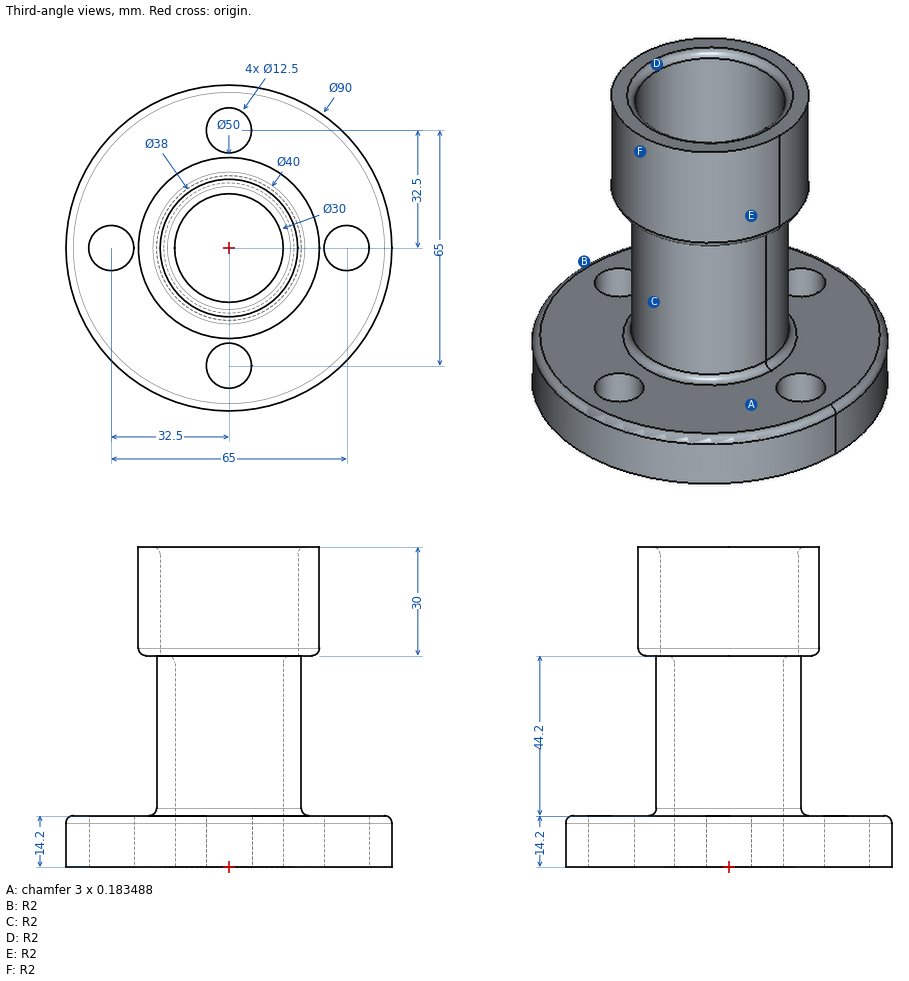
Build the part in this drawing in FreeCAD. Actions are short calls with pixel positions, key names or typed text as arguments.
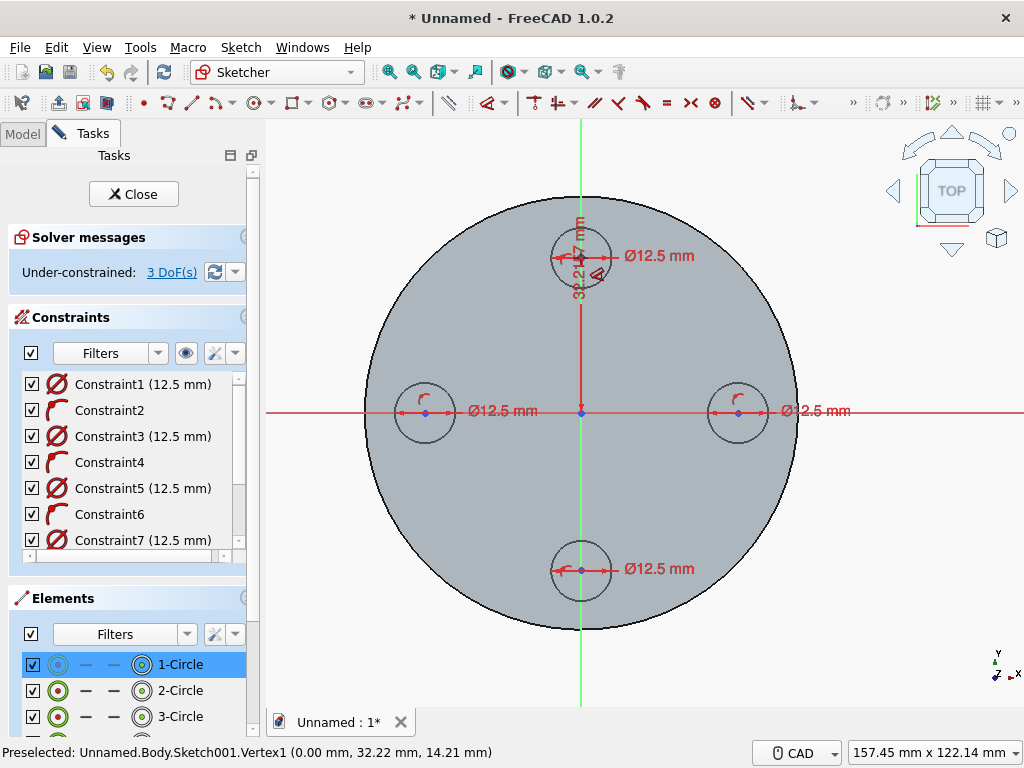
click(581, 571)
click(615, 343)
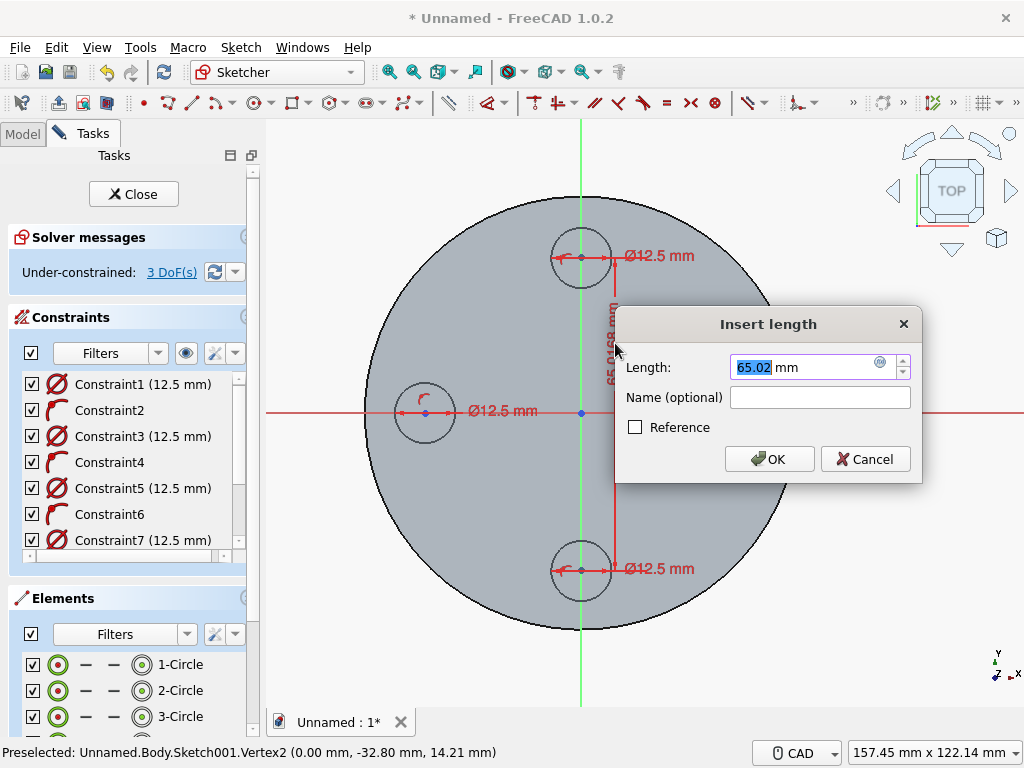
text(65)
key(Return)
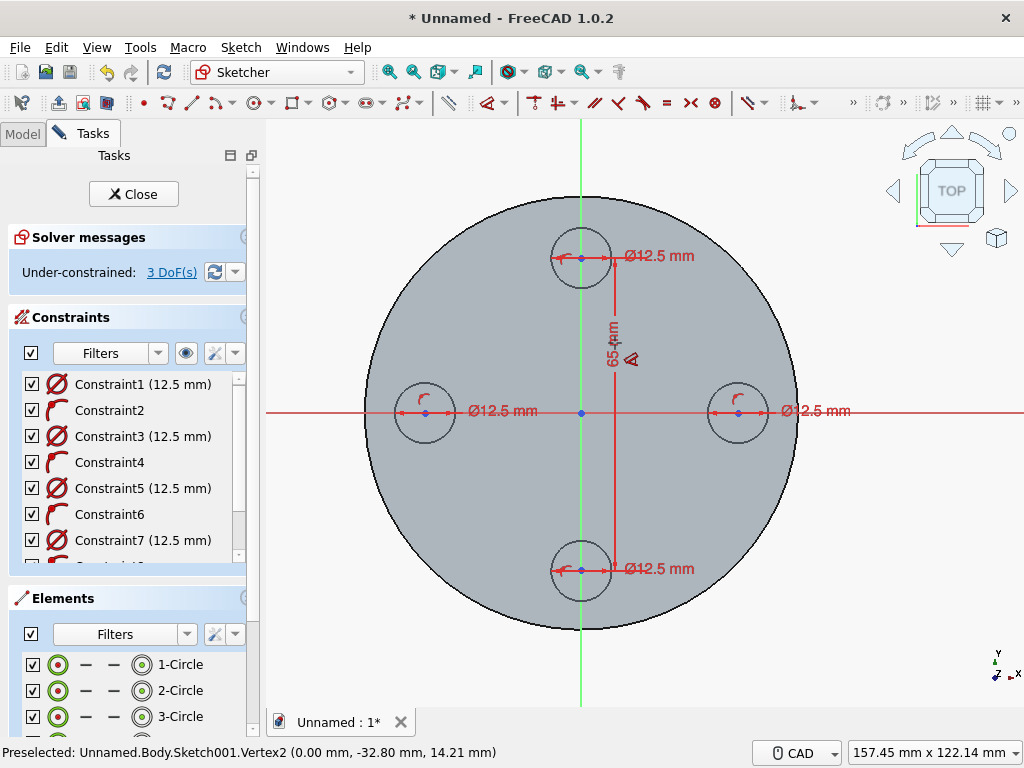
click(425, 413)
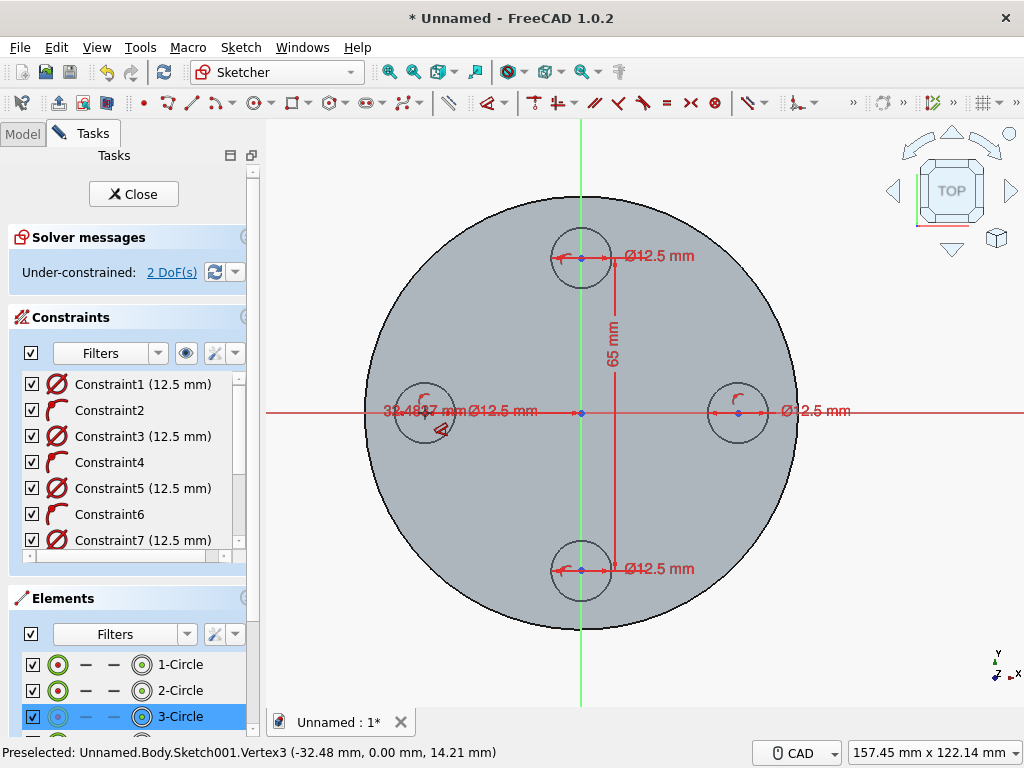
click(738, 413)
click(510, 447)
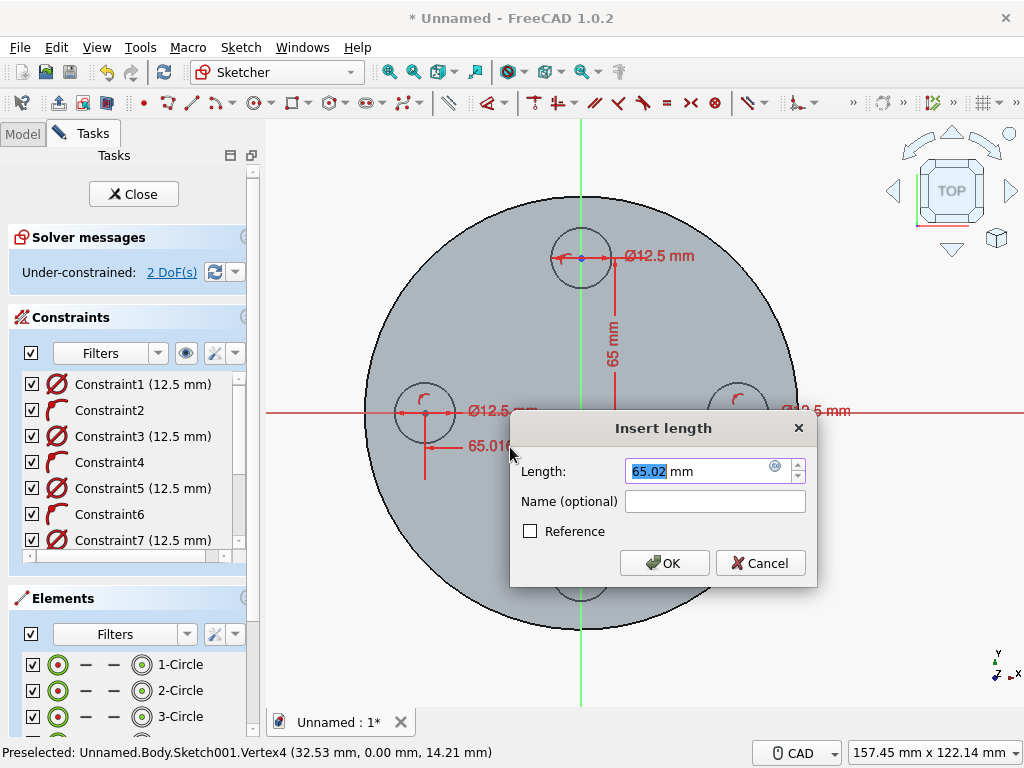
text(65)
key(Return)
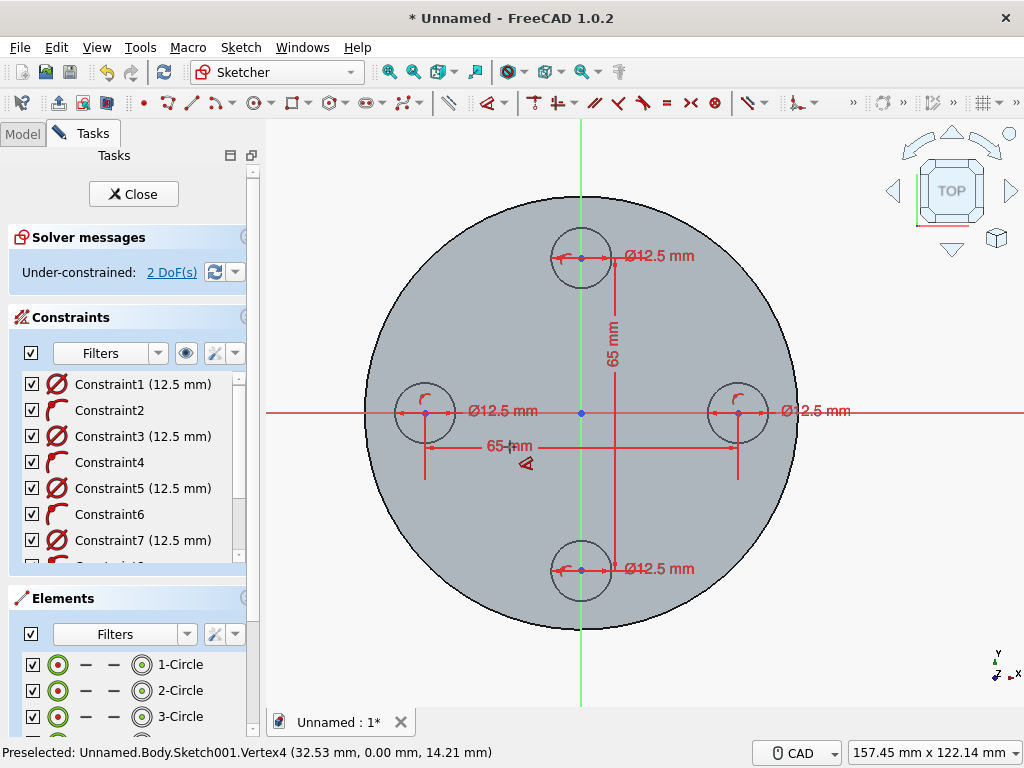
click(581, 258)
click(615, 300)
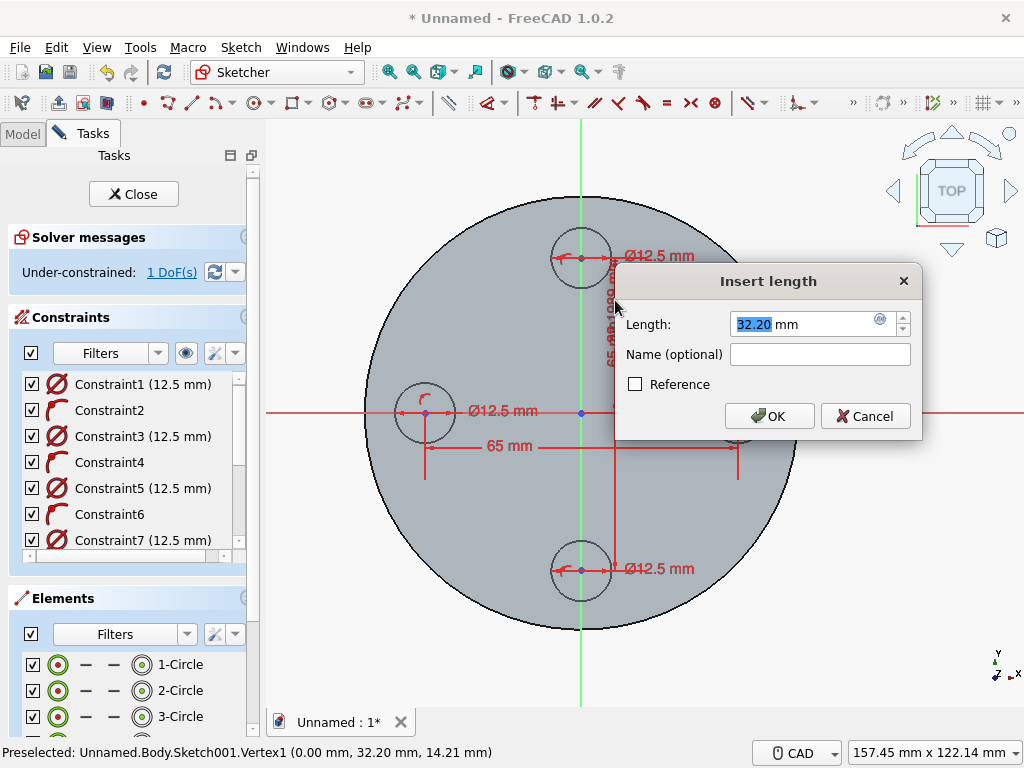
text(32.5)
key(Return)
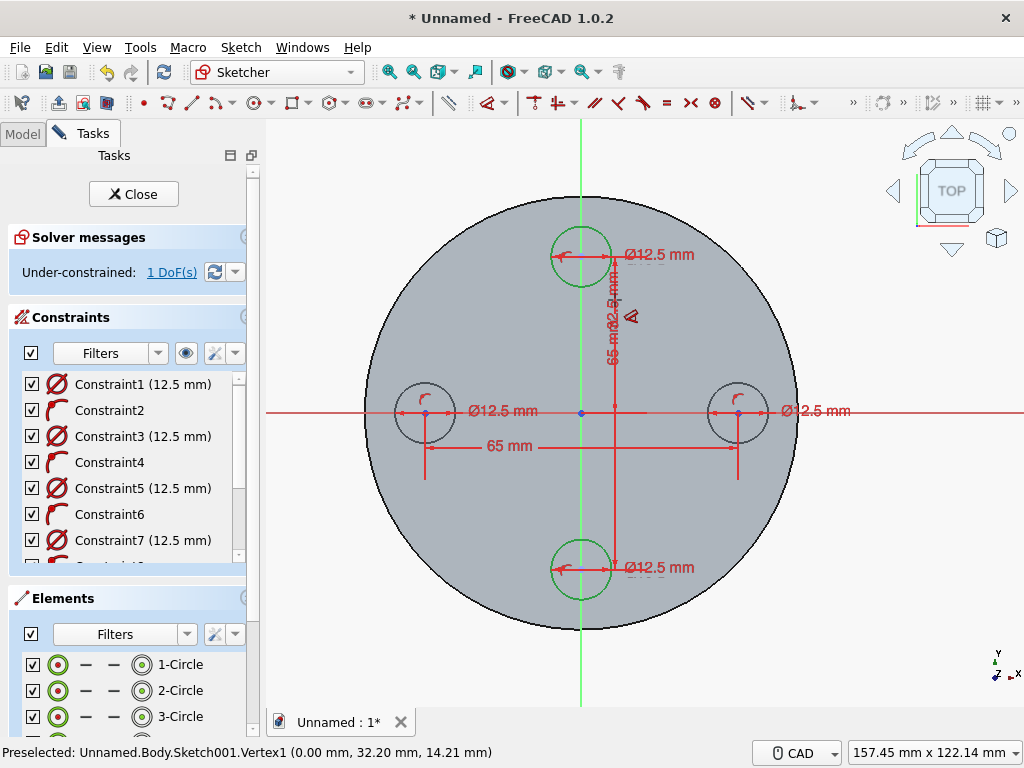
click(425, 413)
click(503, 379)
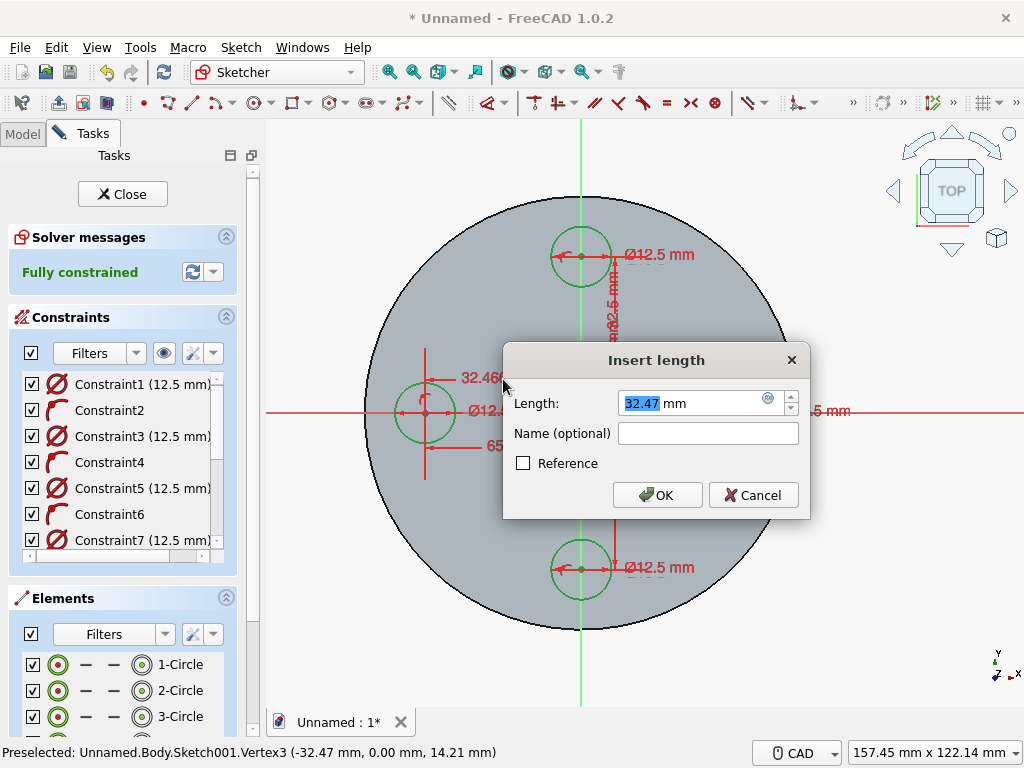
text(32.5)
key(Return)
key(Escape)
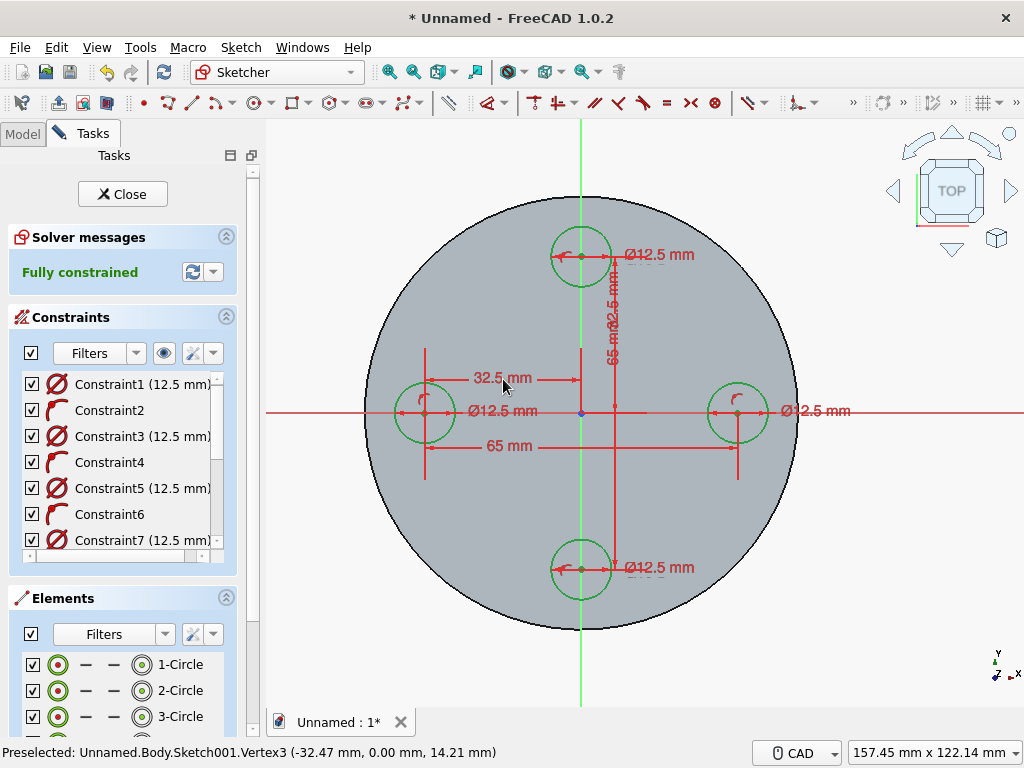
click(123, 194)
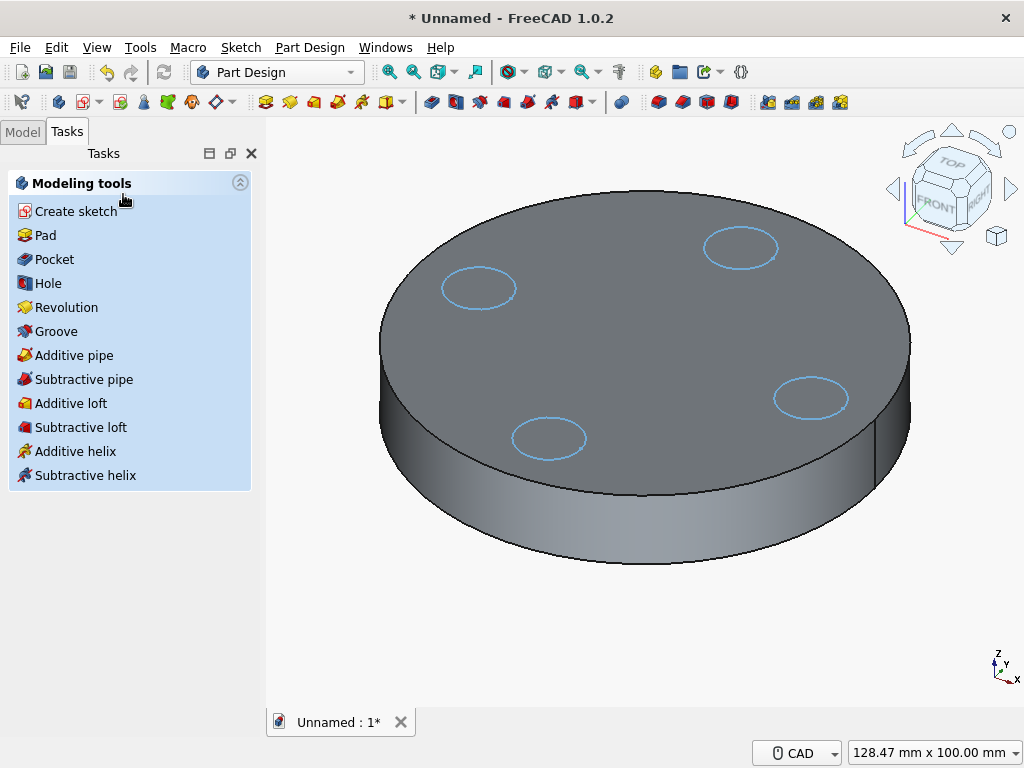
click(432, 102)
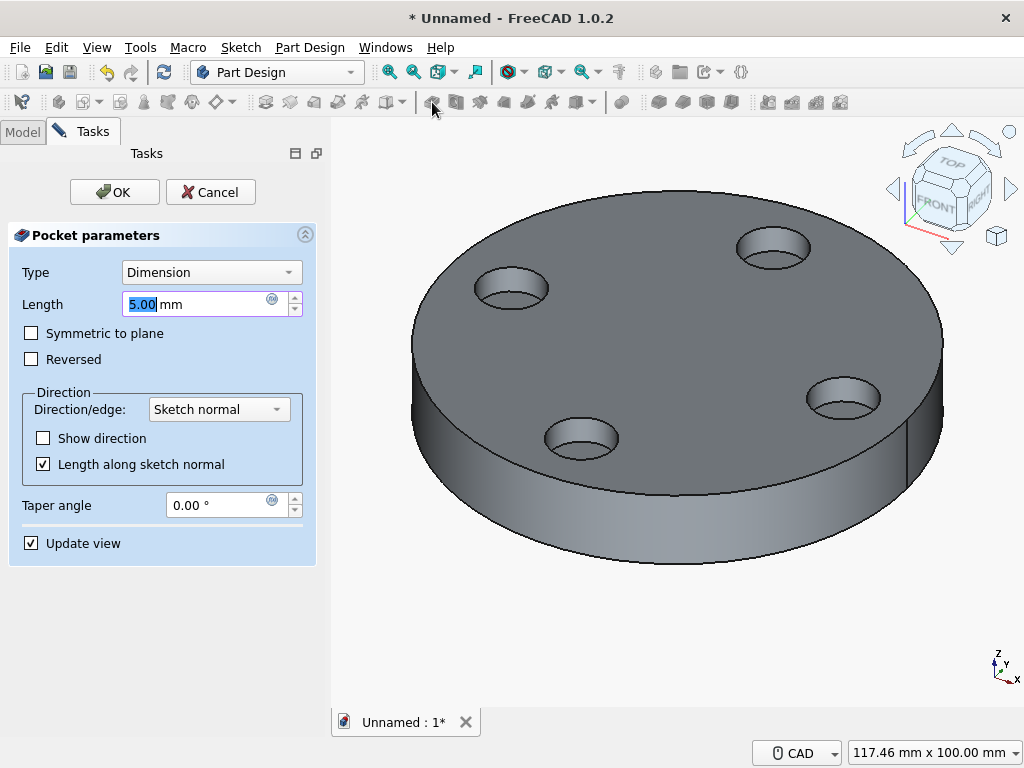
text(14.2)
key(Tab)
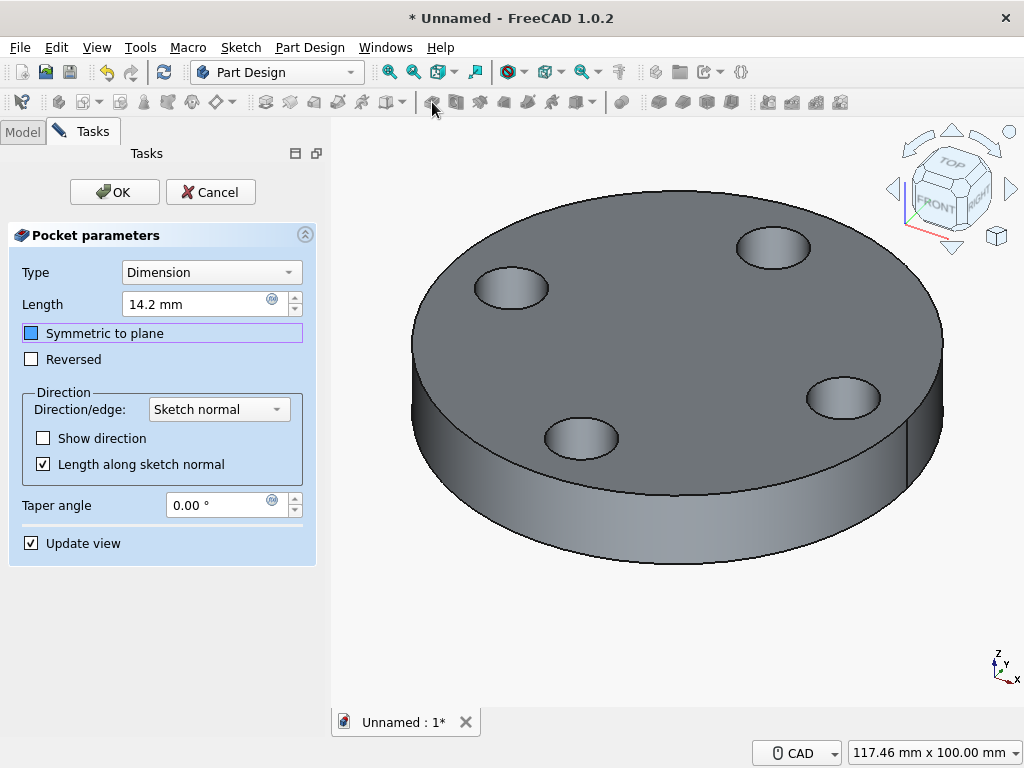
click(115, 192)